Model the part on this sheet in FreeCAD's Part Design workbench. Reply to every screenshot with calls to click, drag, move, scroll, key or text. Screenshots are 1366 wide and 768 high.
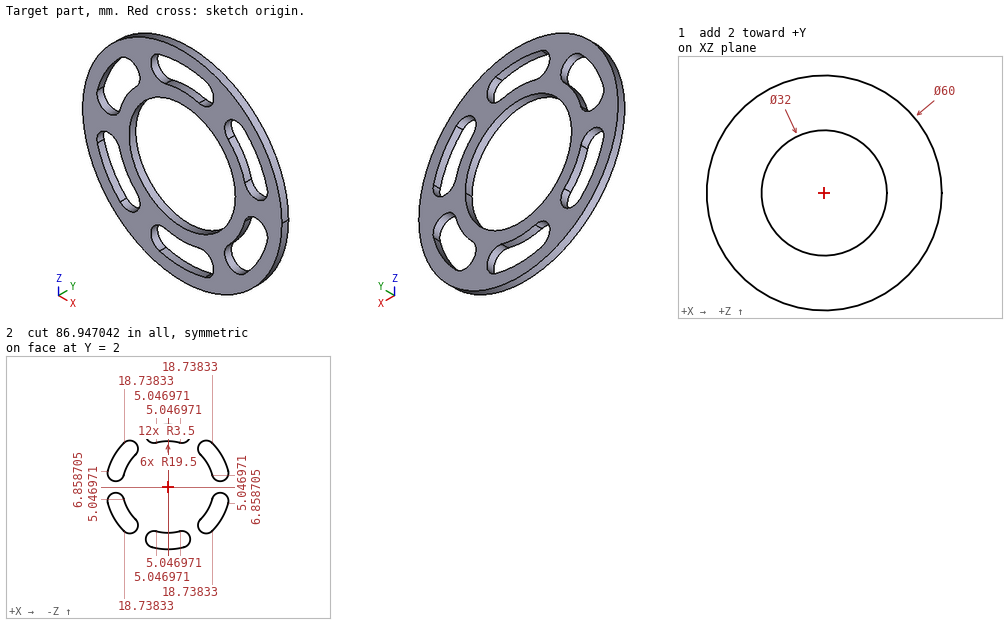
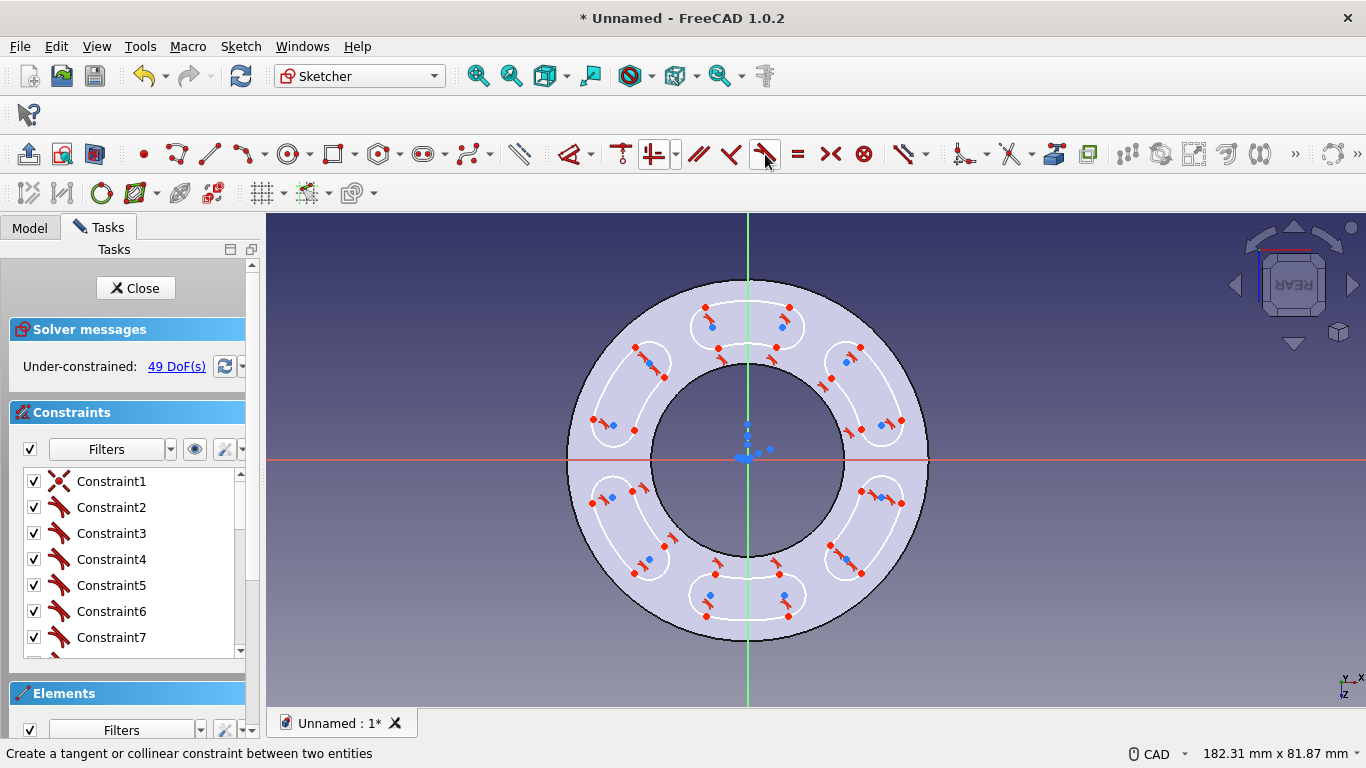
click(597, 439)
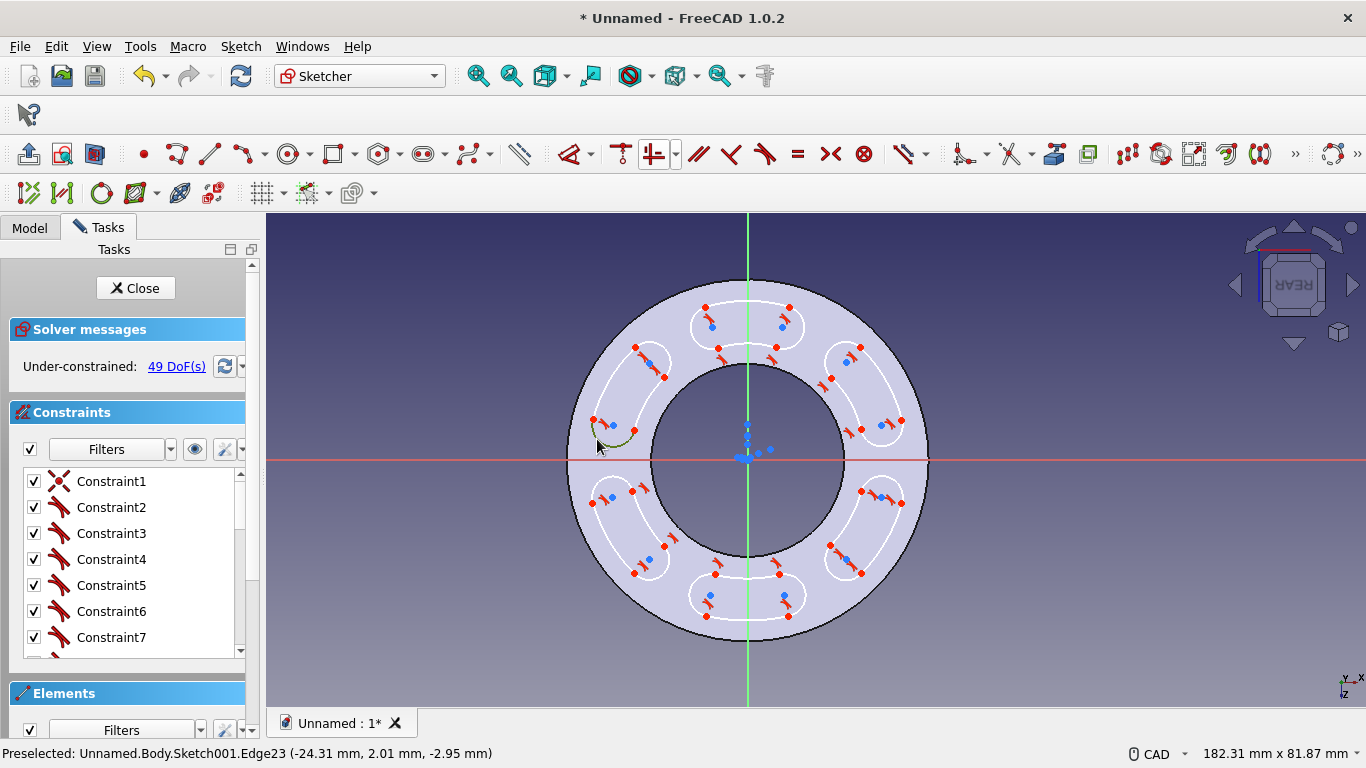
click(652, 392)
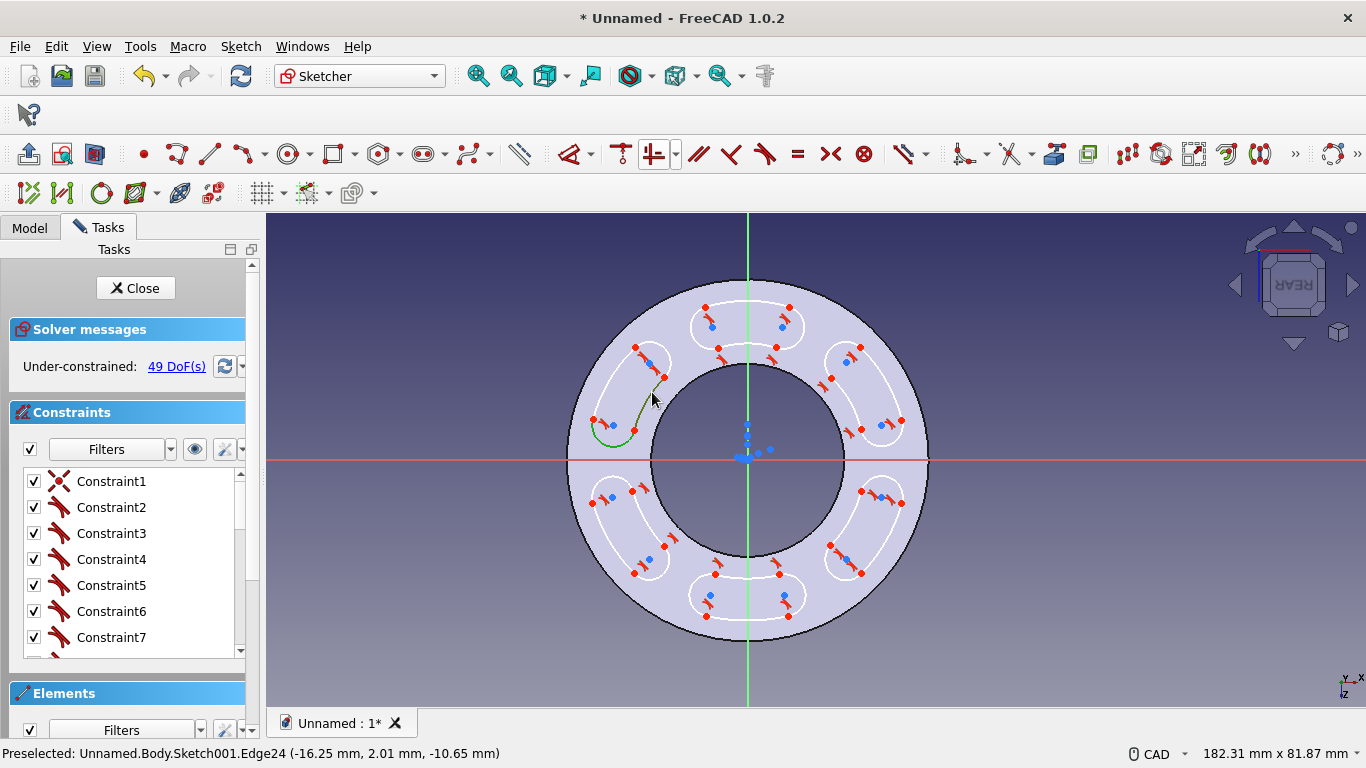
click(765, 154)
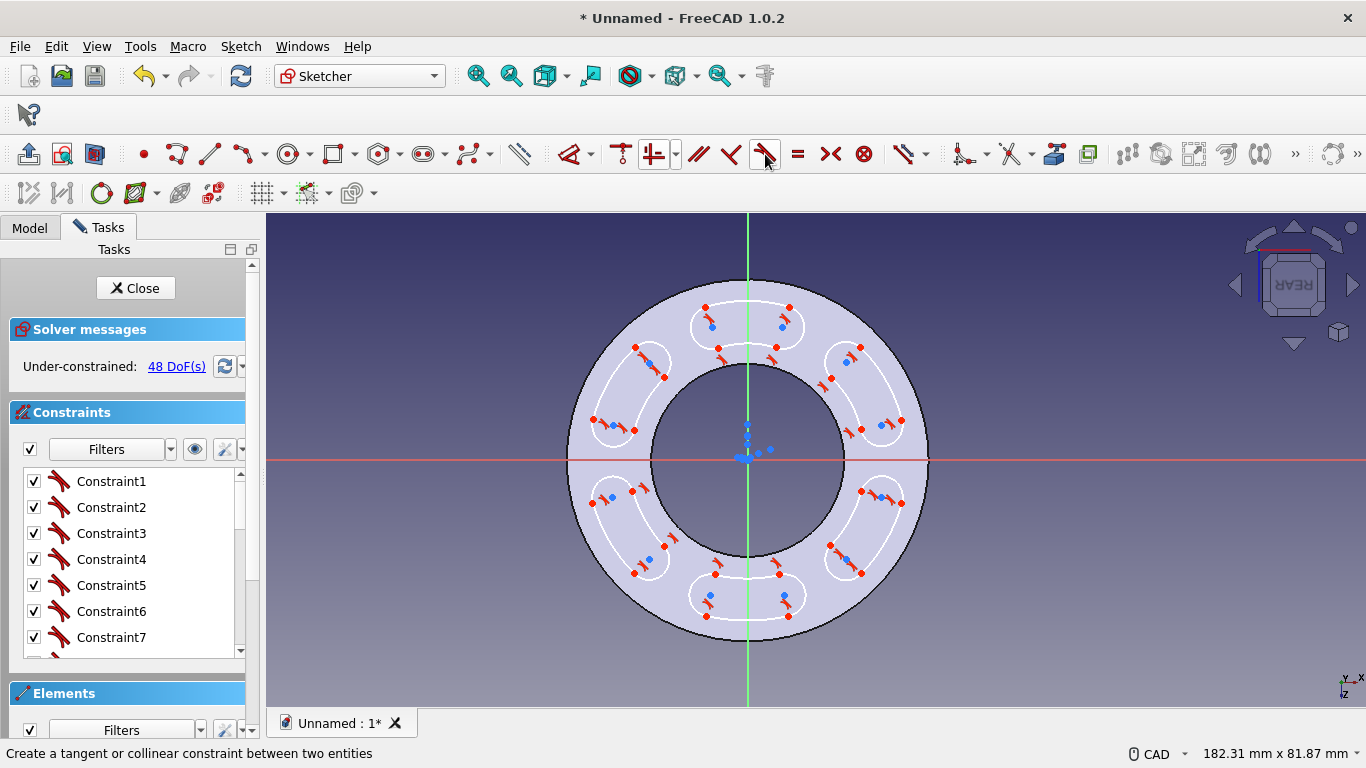
click(759, 344)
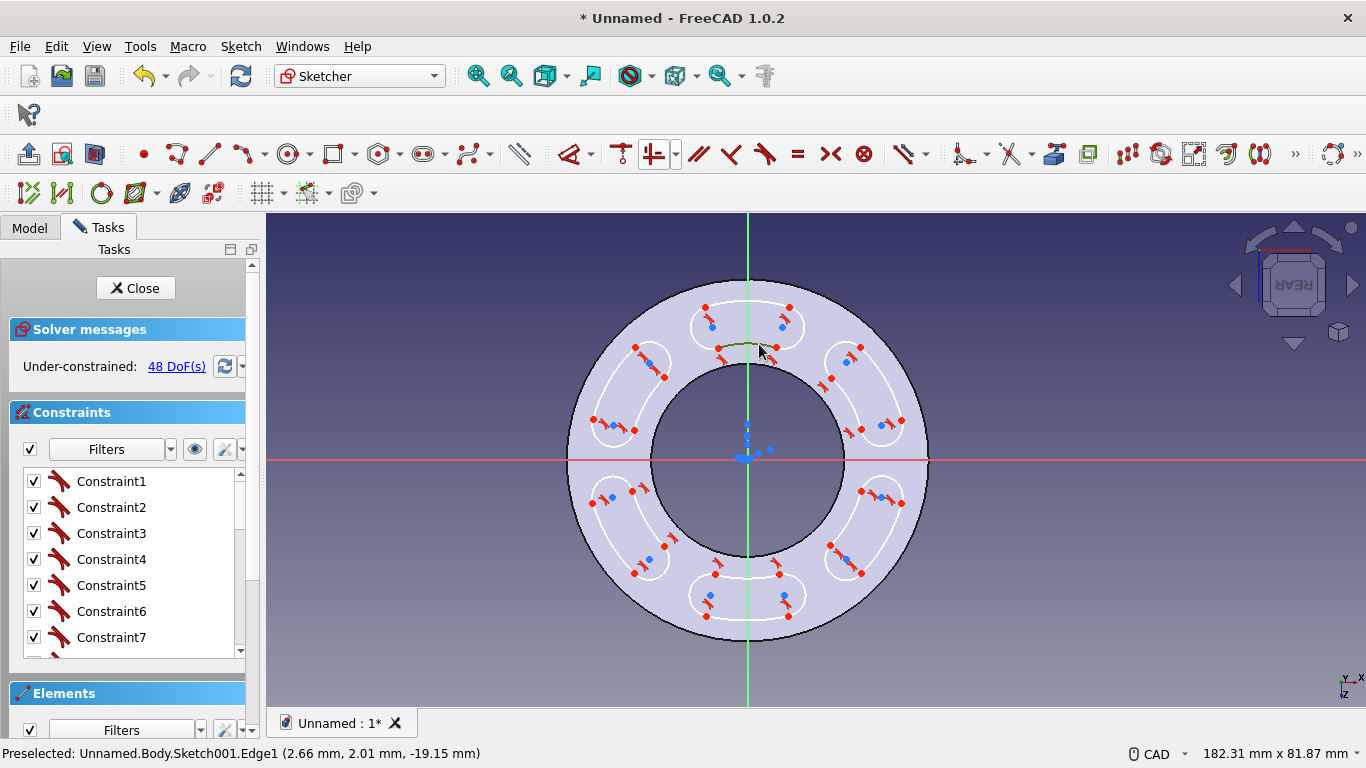
click(764, 302)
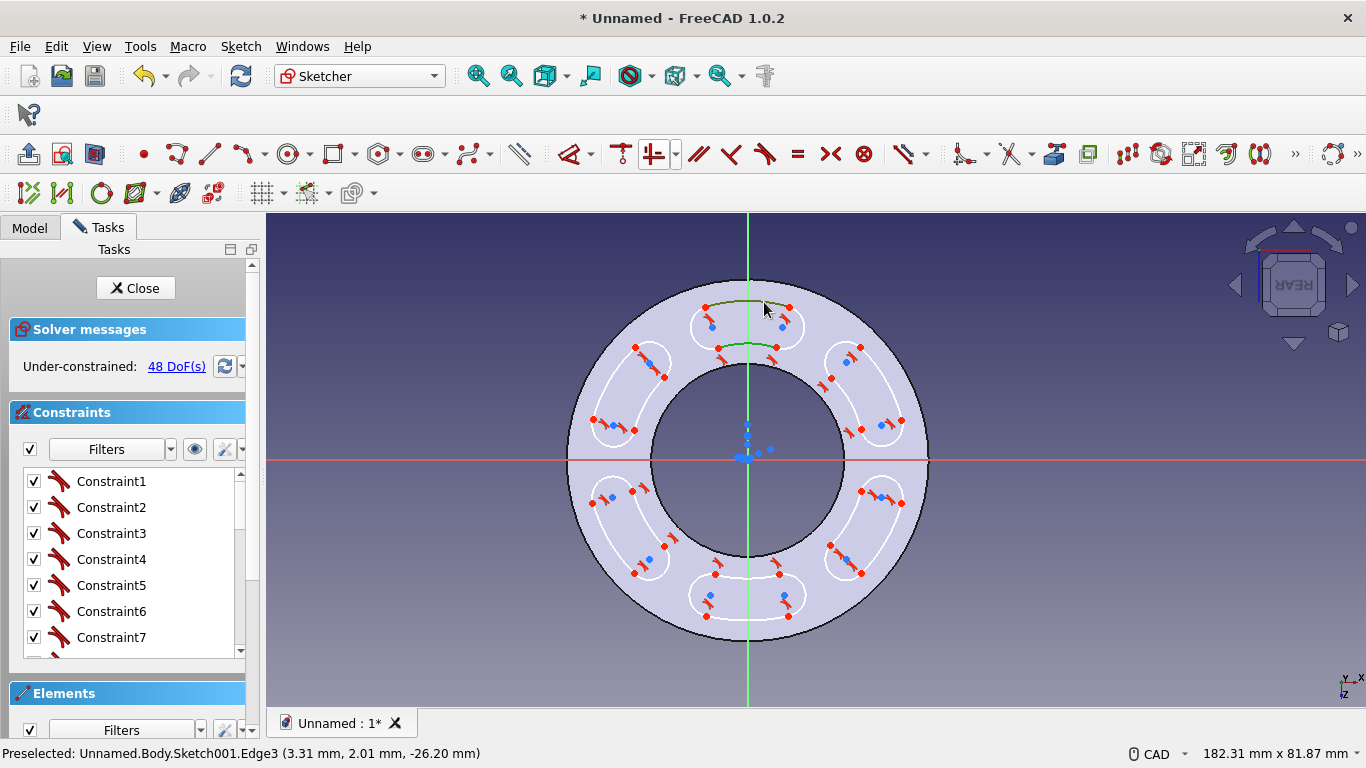
key(c)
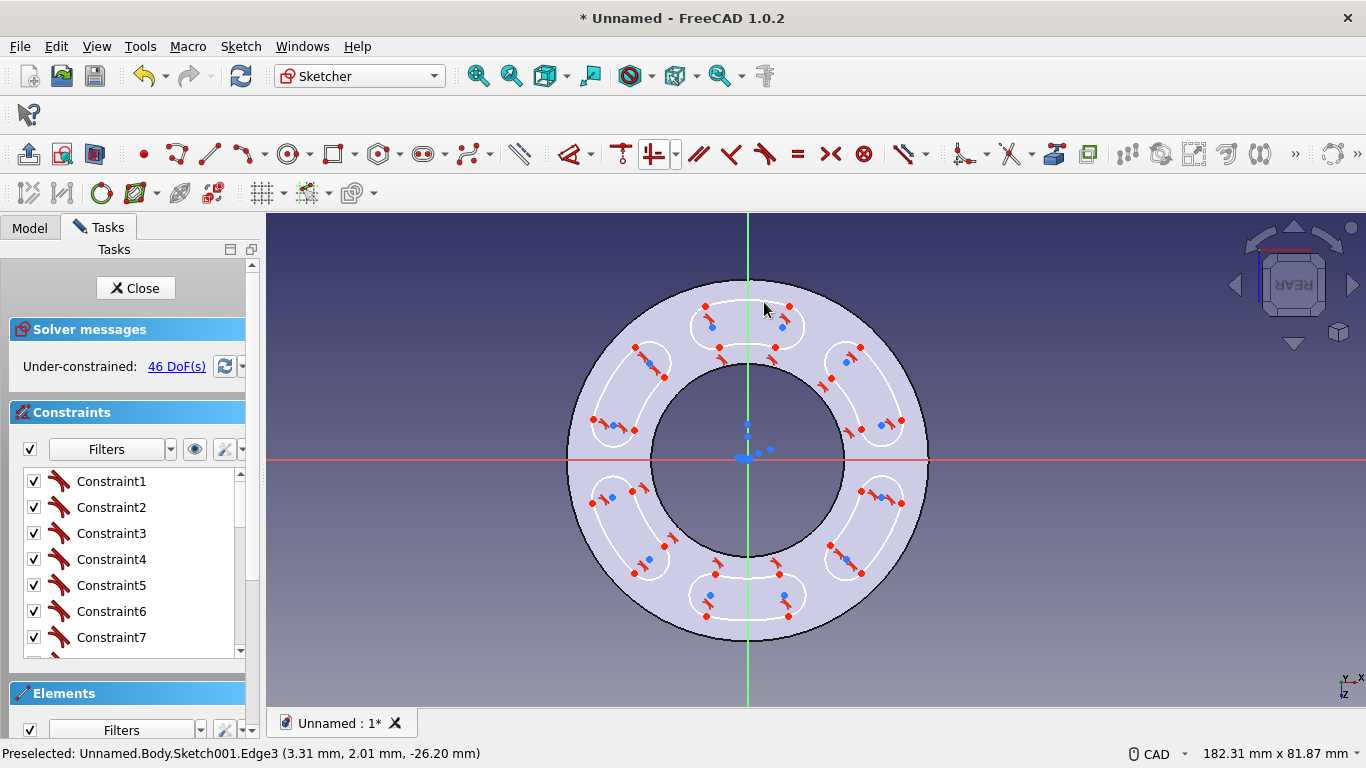
click(759, 344)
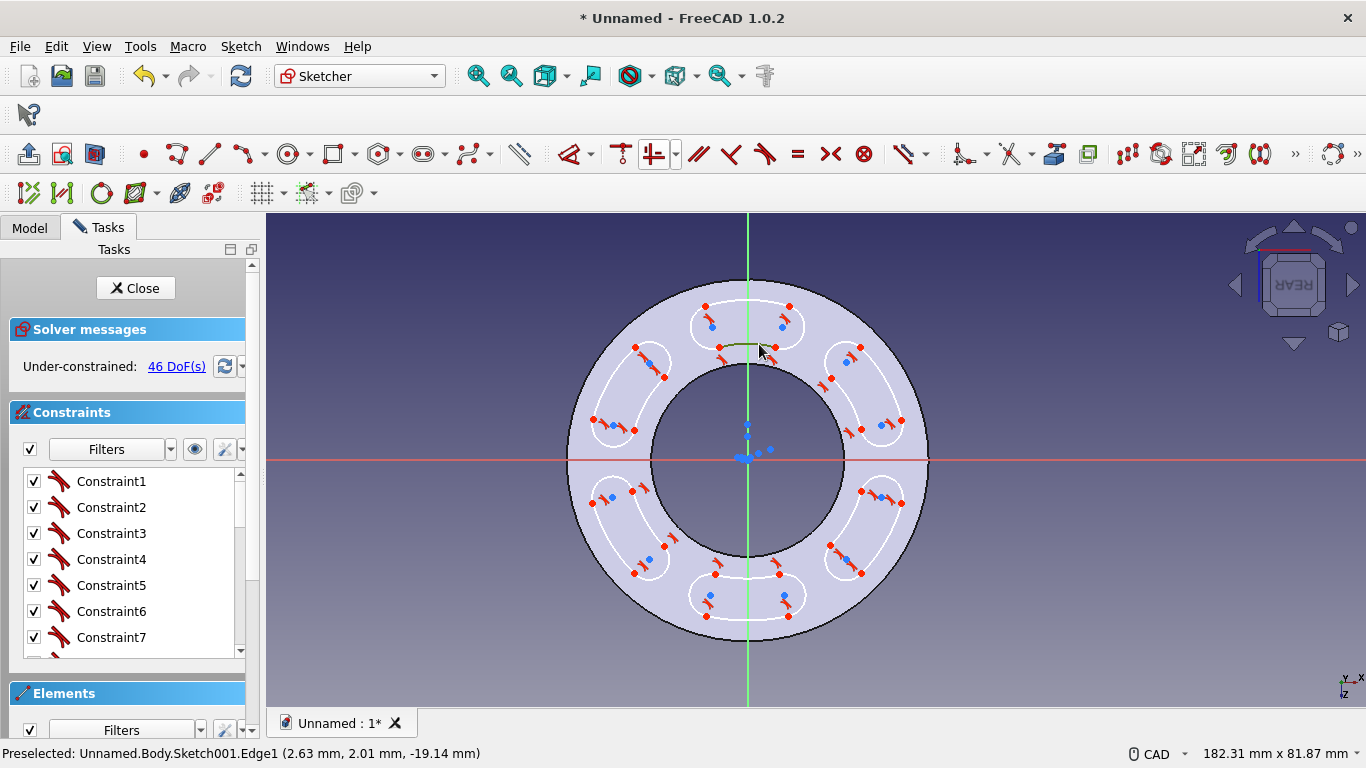
click(856, 413)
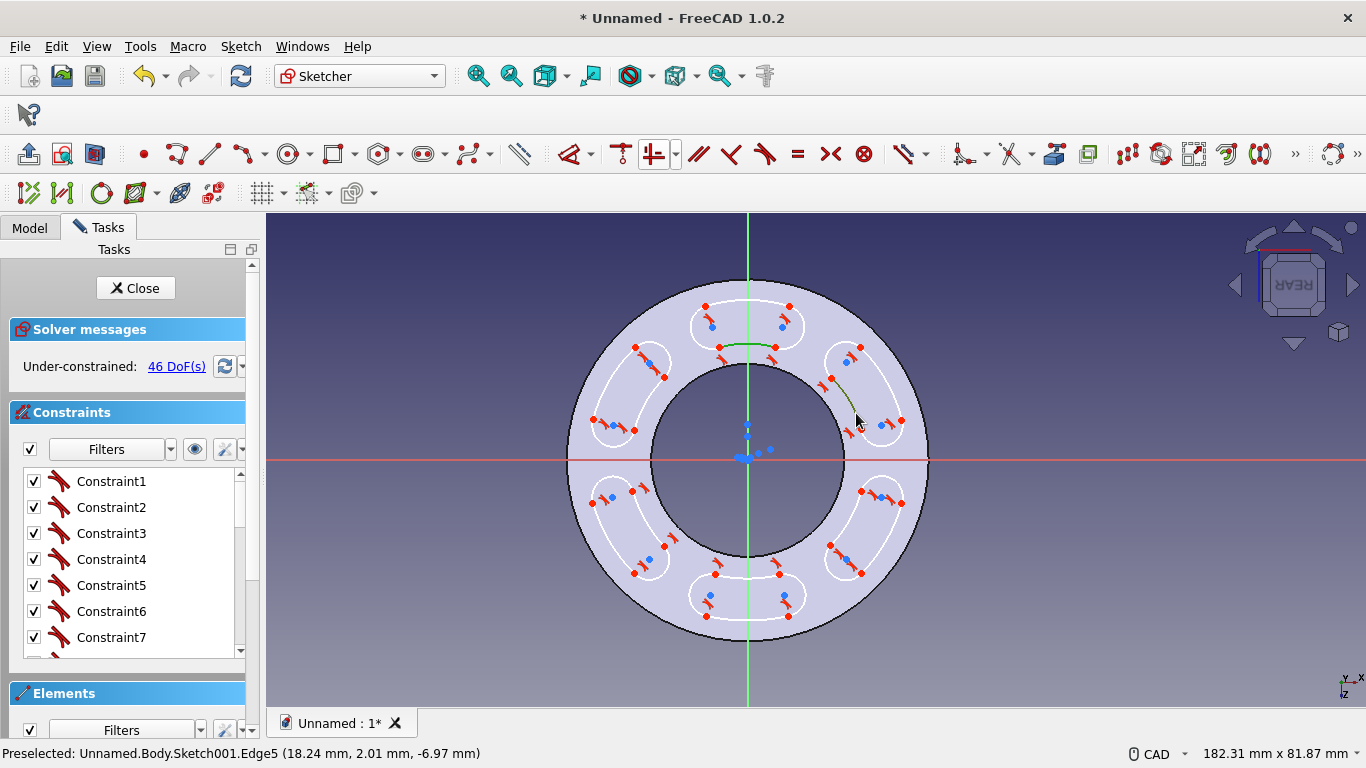
click(621, 154)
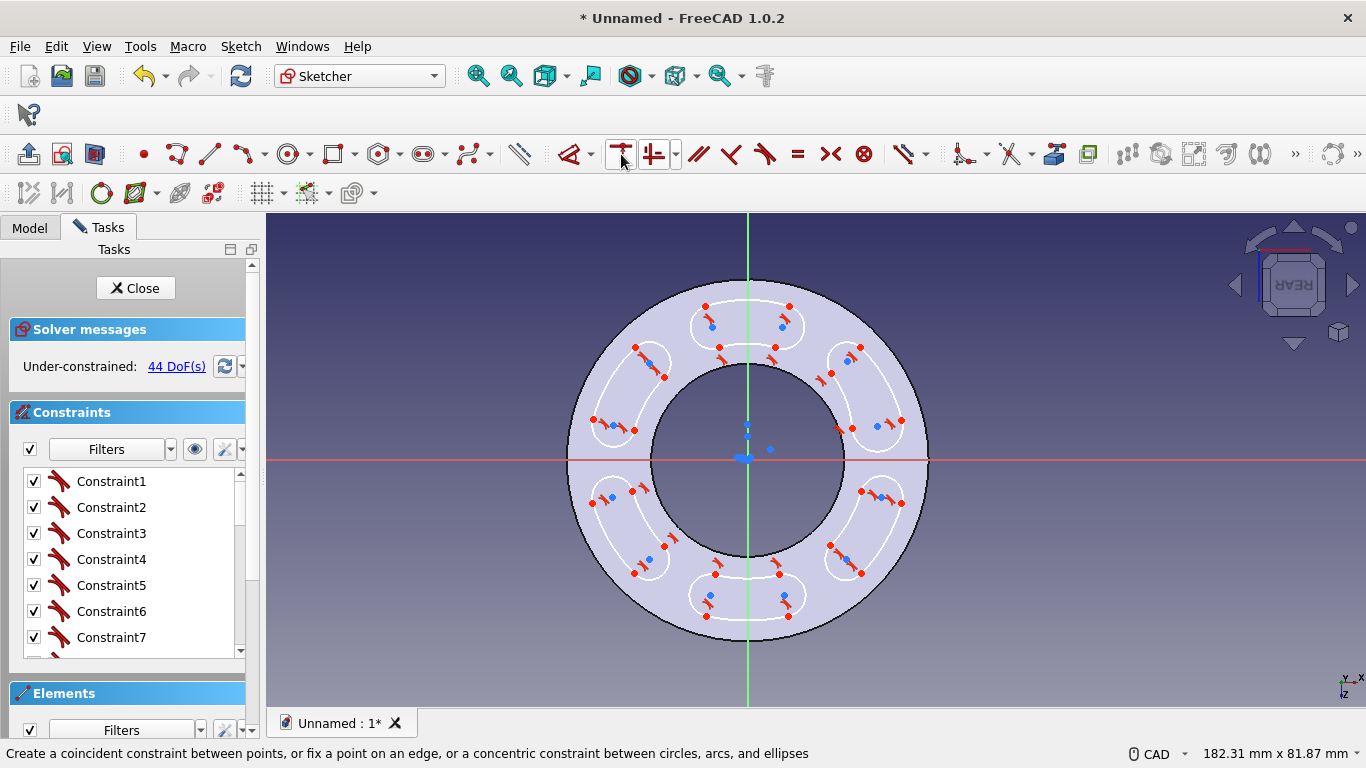
click(759, 344)